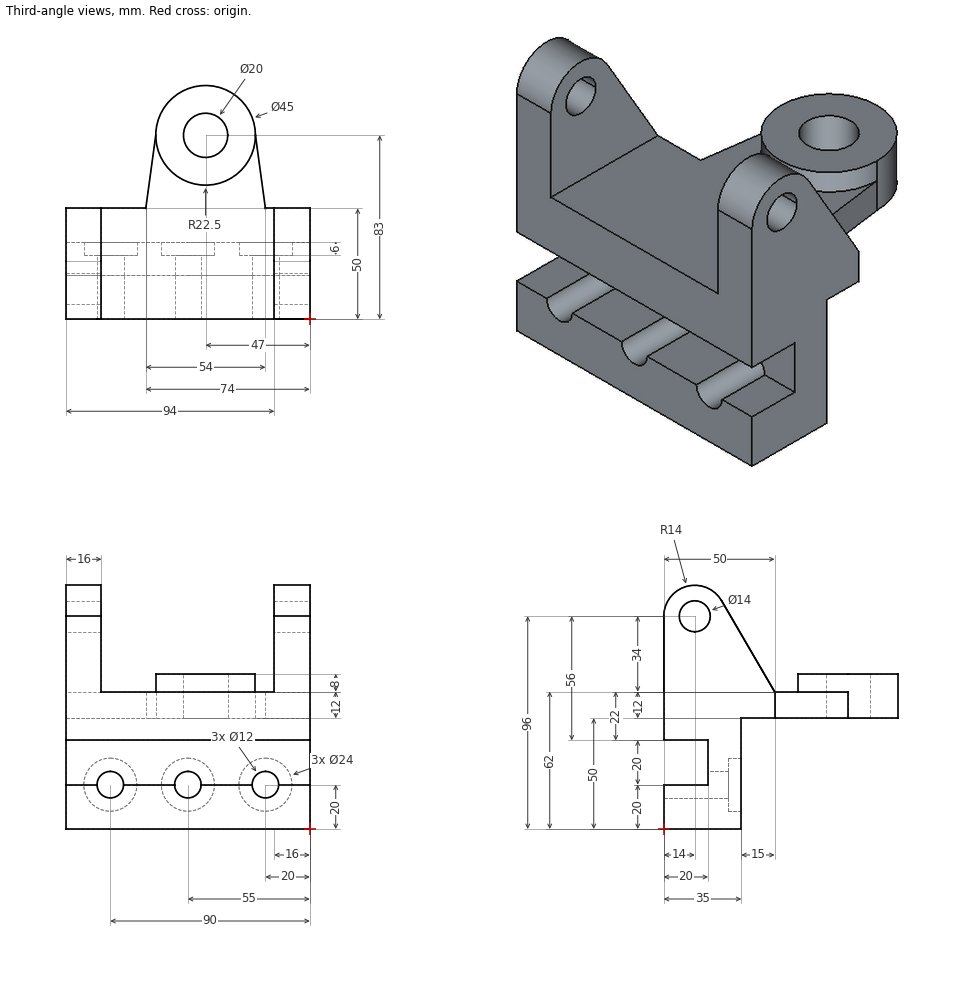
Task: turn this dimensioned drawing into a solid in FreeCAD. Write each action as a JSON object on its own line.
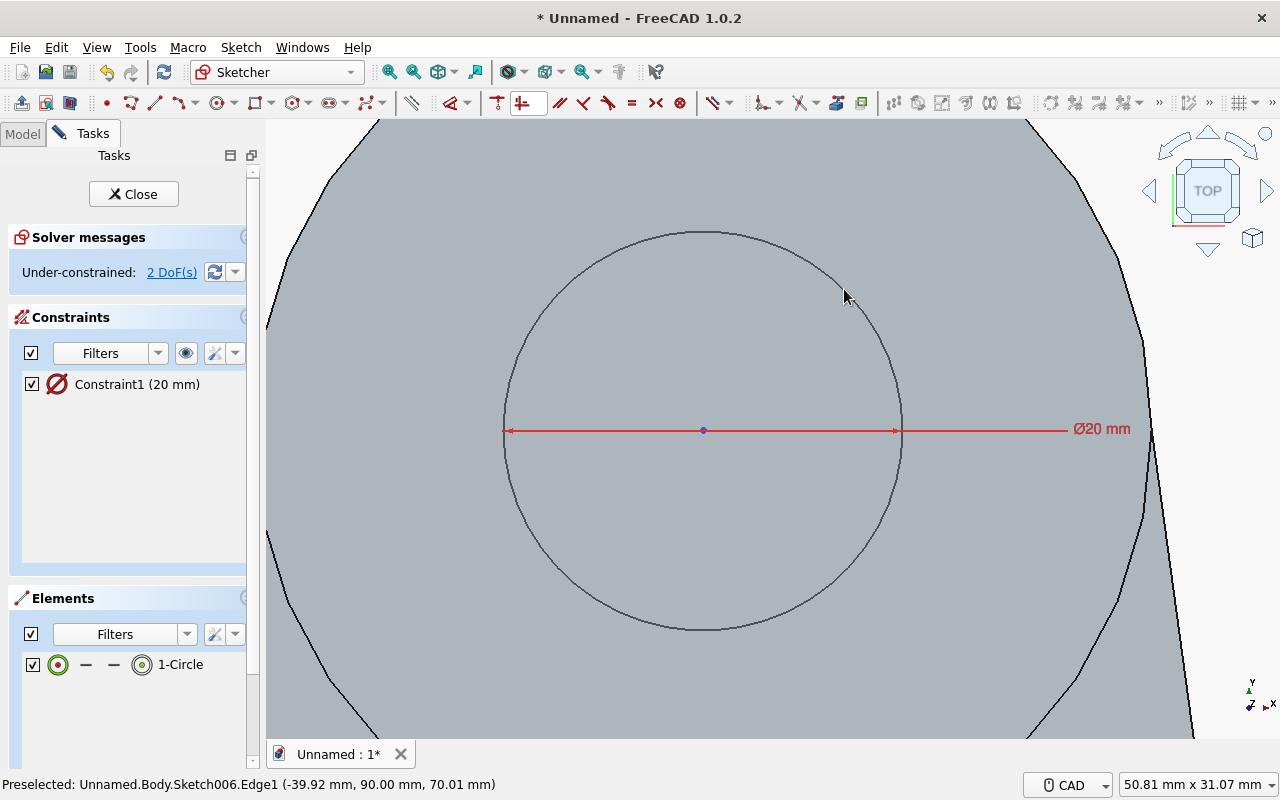
{"action": "left_click", "coordinate": [450, 104]}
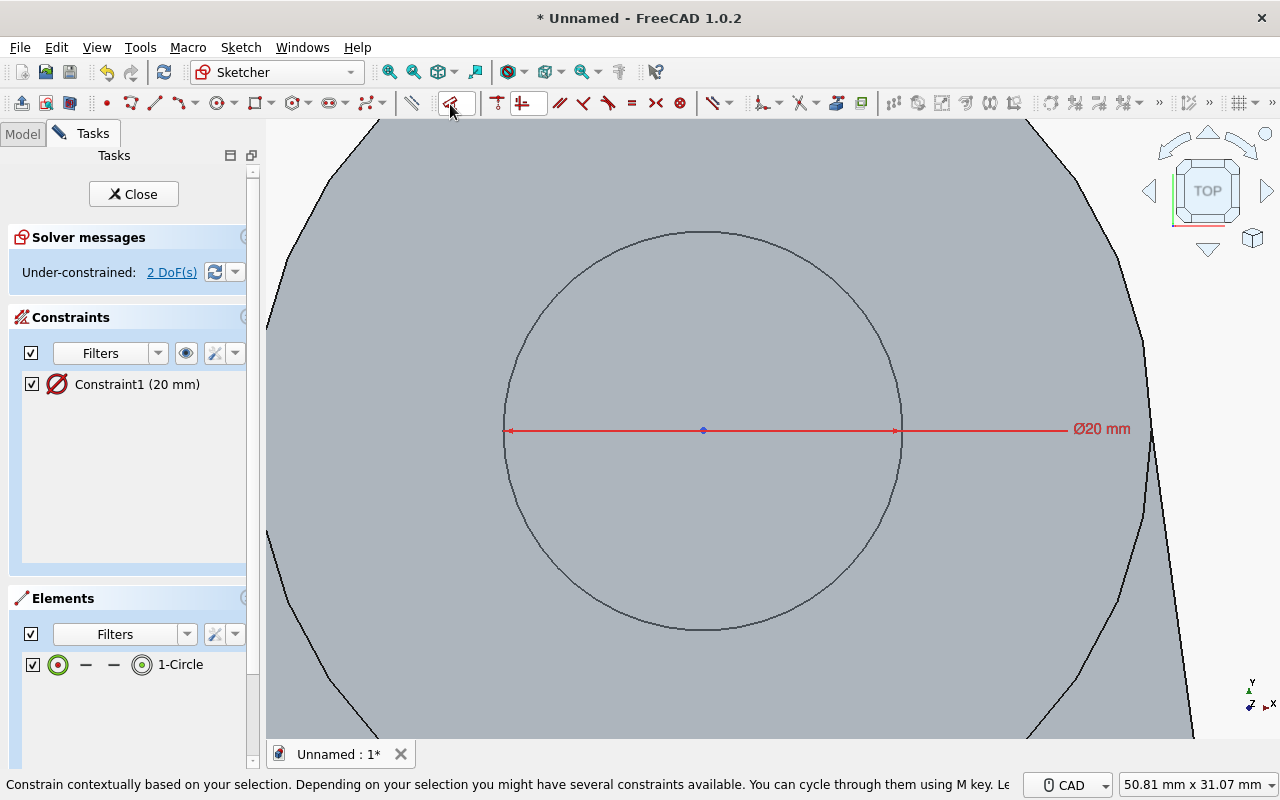
{"action": "left_click", "coordinate": [703, 431]}
{"action": "left_click", "coordinate": [814, 397]}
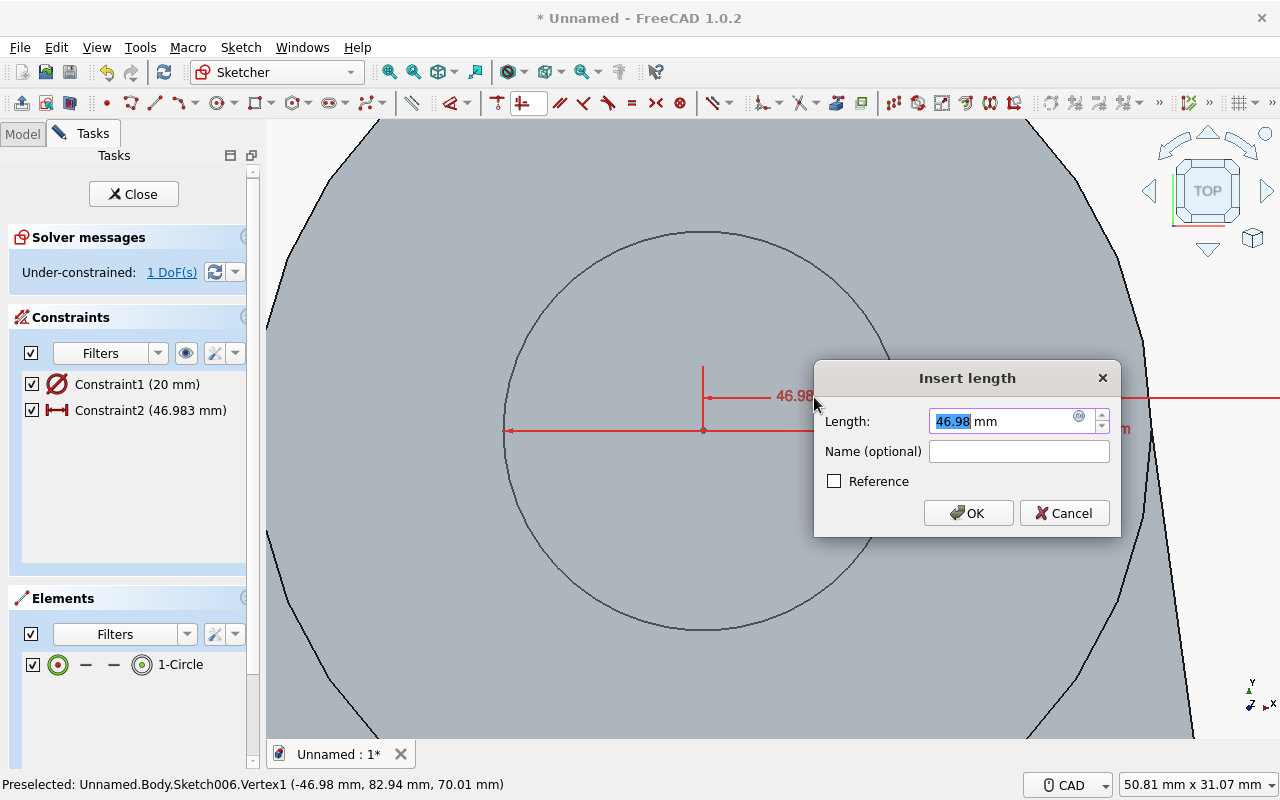
{"action": "type", "text": "47"}
{"action": "key", "text": "Return"}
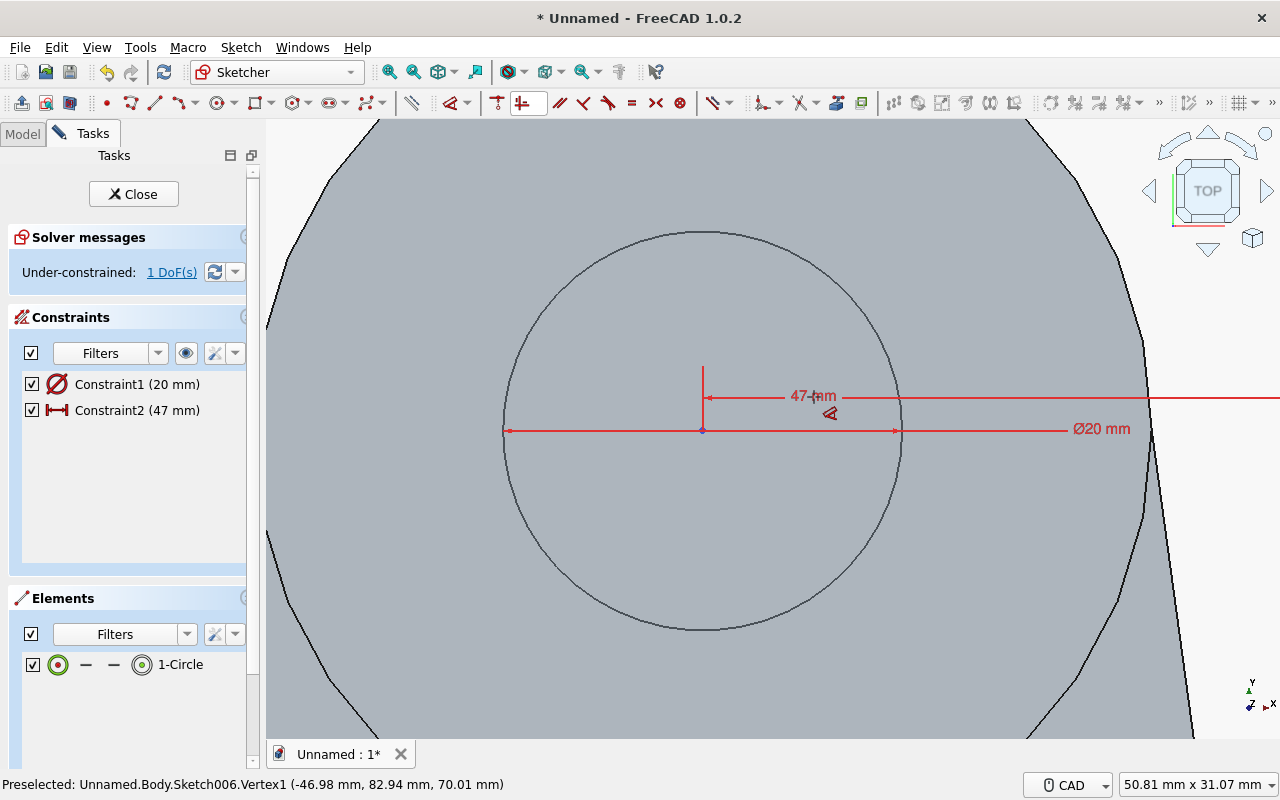
{"action": "left_click", "coordinate": [703, 431]}
{"action": "left_click", "coordinate": [669, 571]}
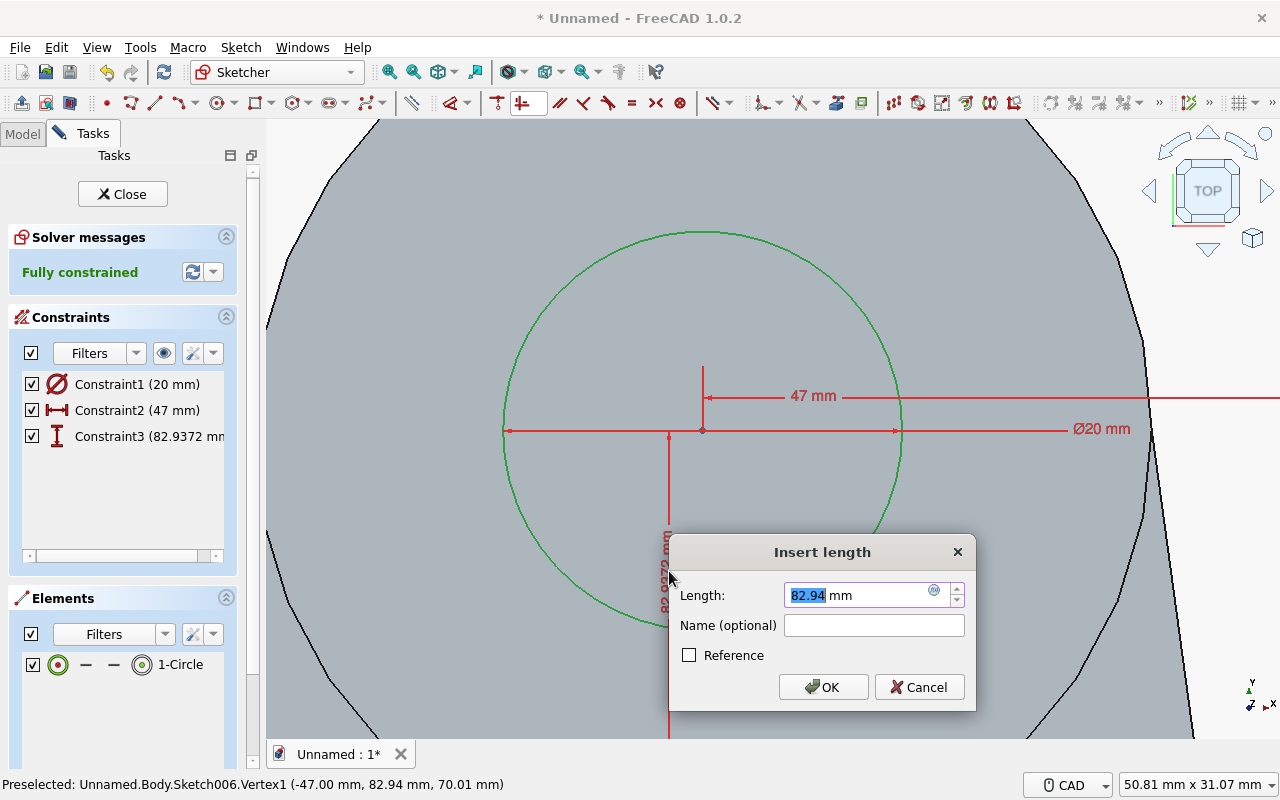
{"action": "type", "text": "83"}
{"action": "key", "text": "Return"}
{"action": "key", "text": "Escape"}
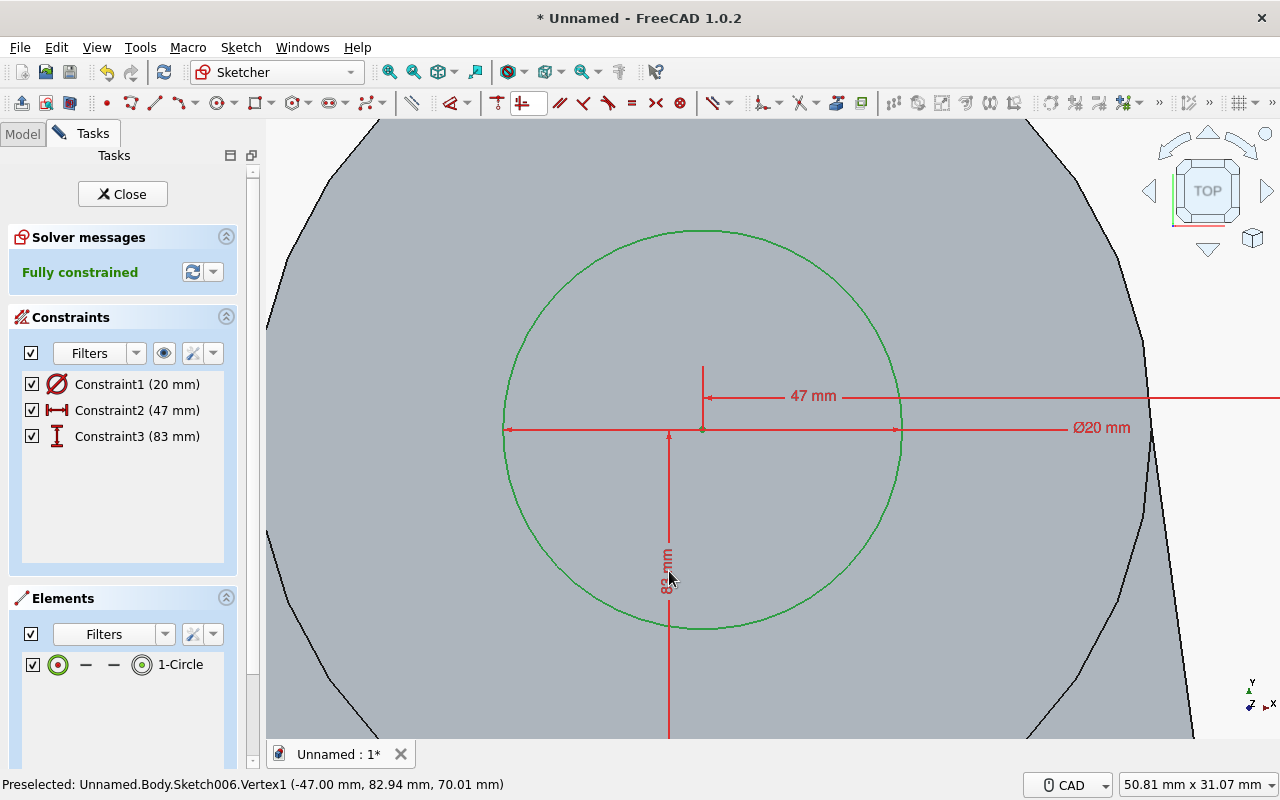
{"action": "left_click", "coordinate": [123, 194]}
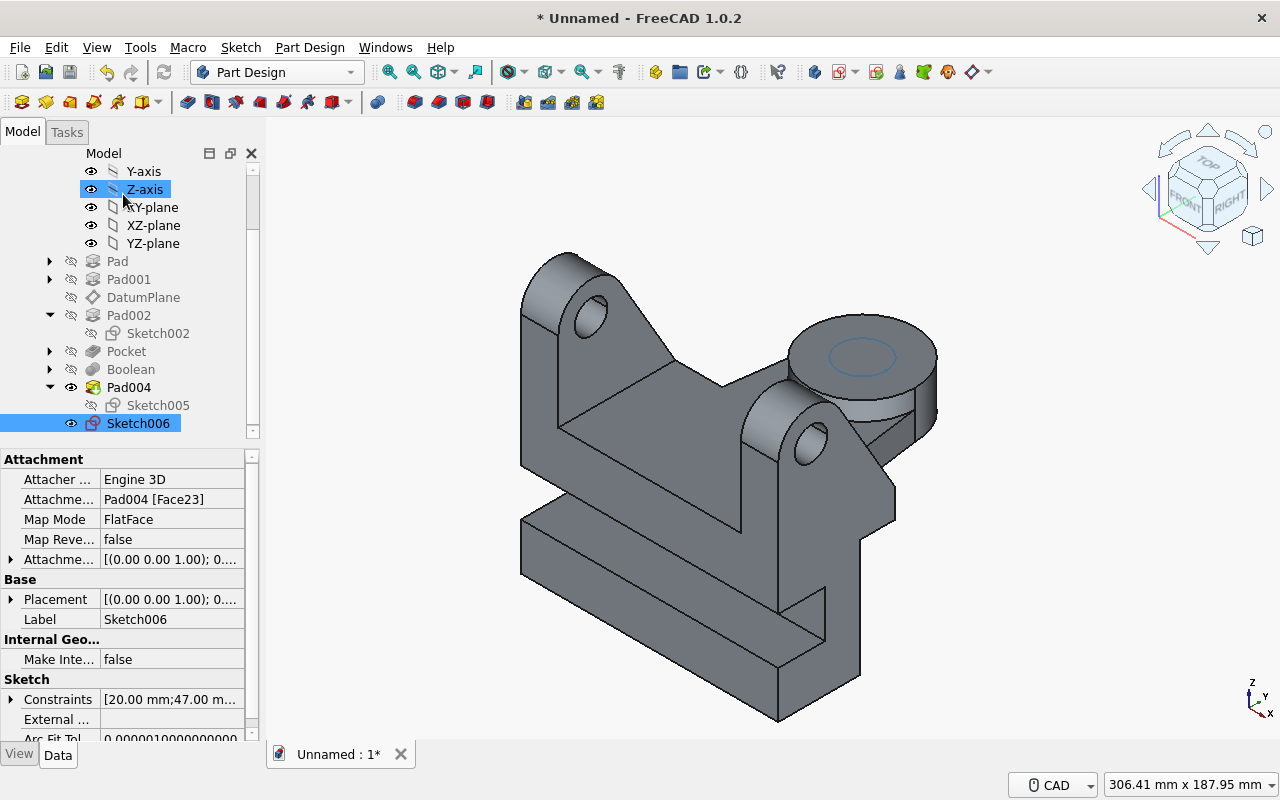
{"action": "left_click", "coordinate": [188, 102]}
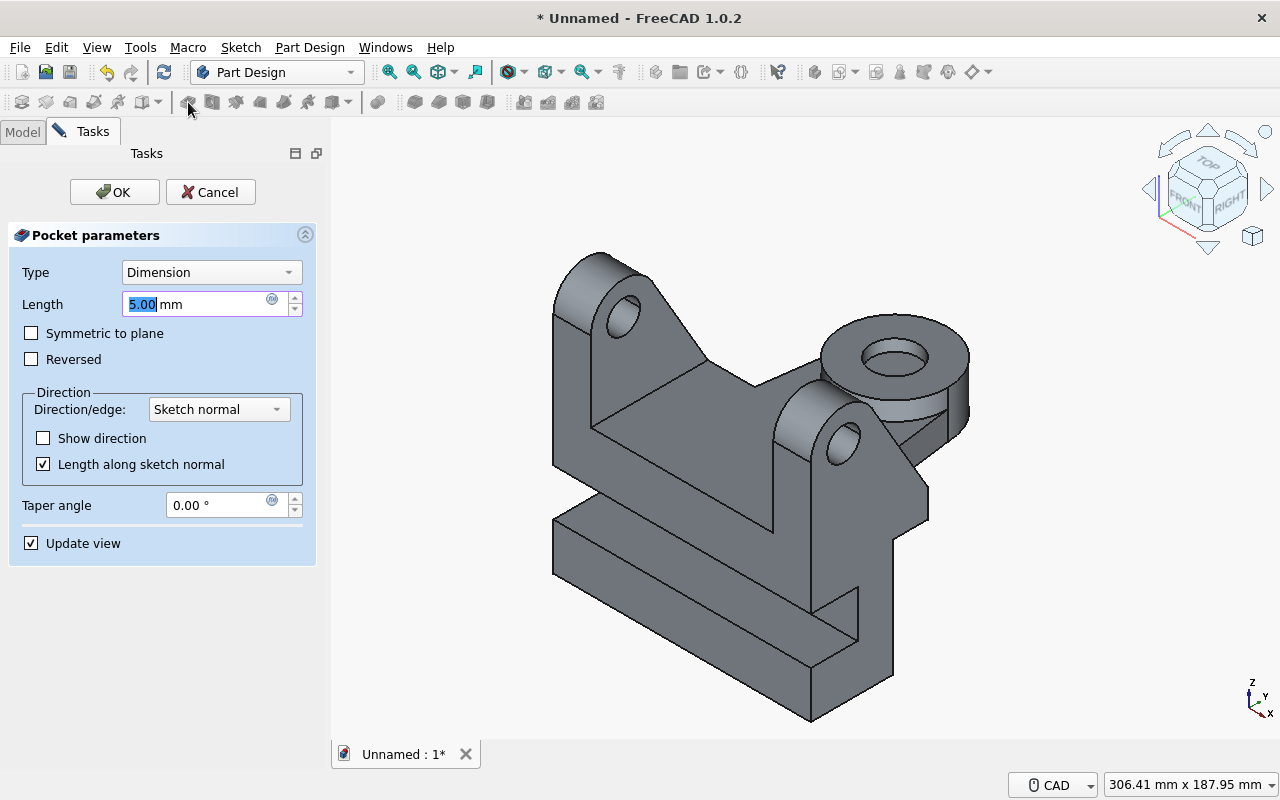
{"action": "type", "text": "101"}
{"action": "key", "text": "Tab"}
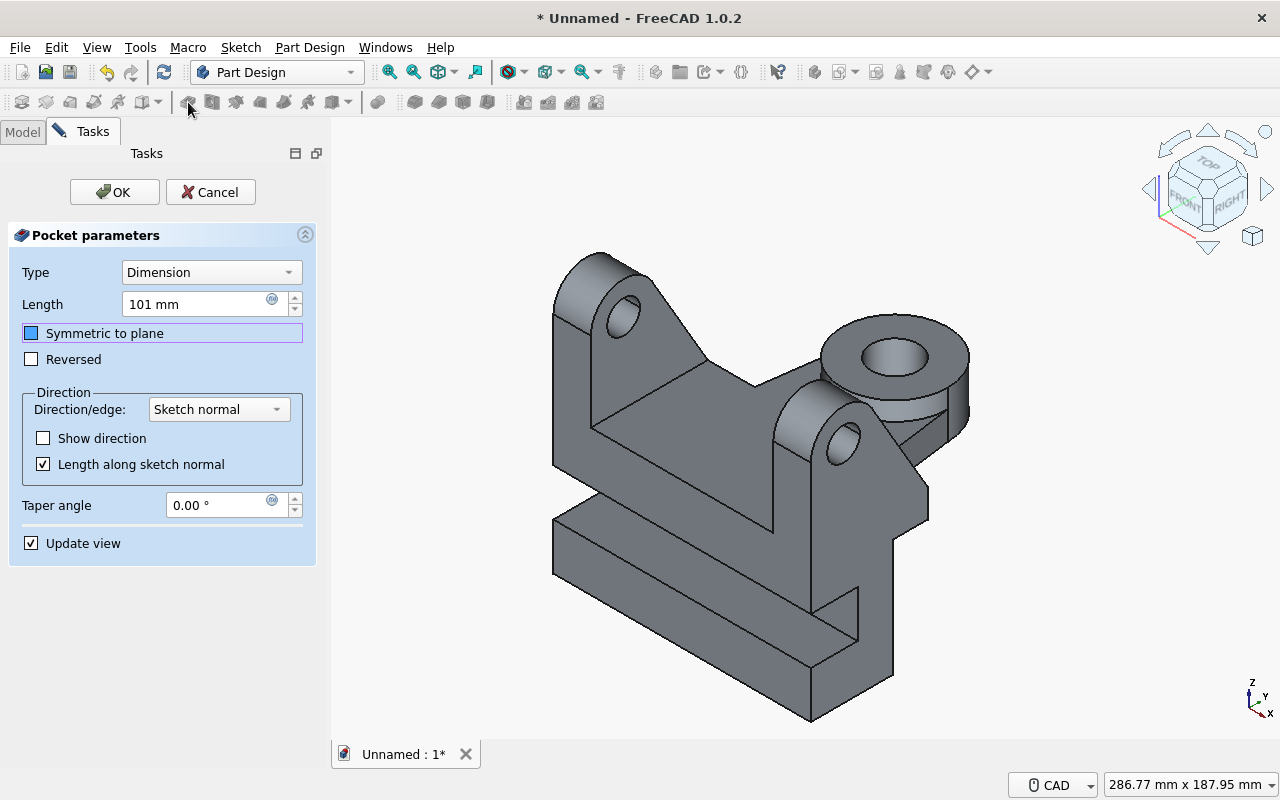
{"action": "left_click", "coordinate": [115, 192]}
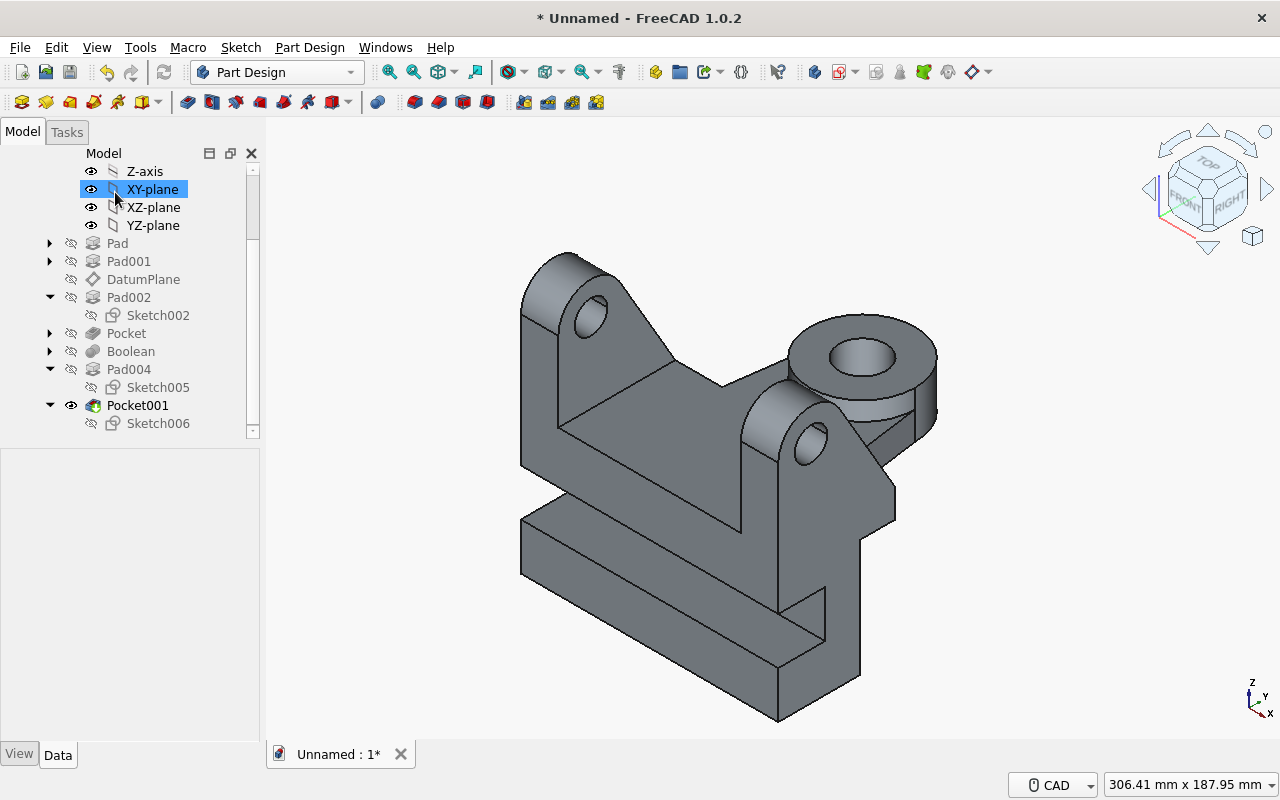
{"action": "key", "text": "4"}